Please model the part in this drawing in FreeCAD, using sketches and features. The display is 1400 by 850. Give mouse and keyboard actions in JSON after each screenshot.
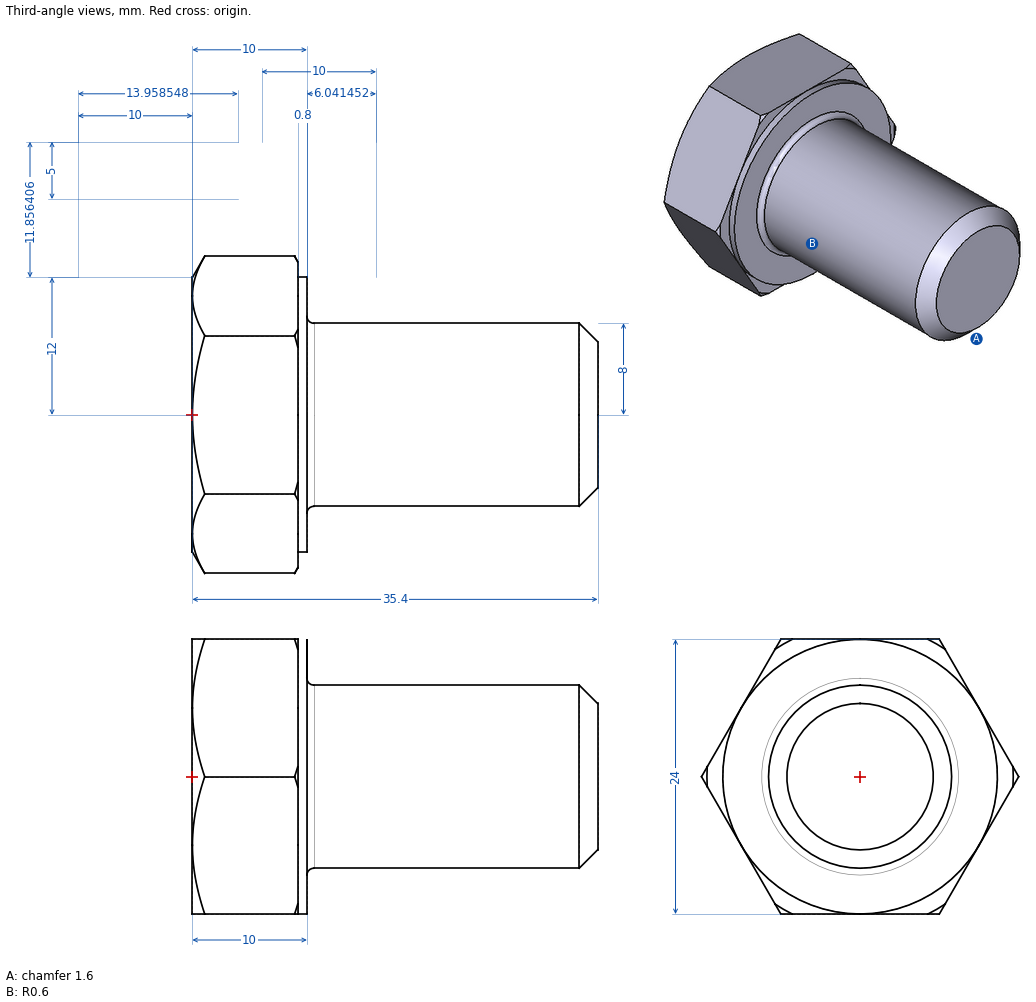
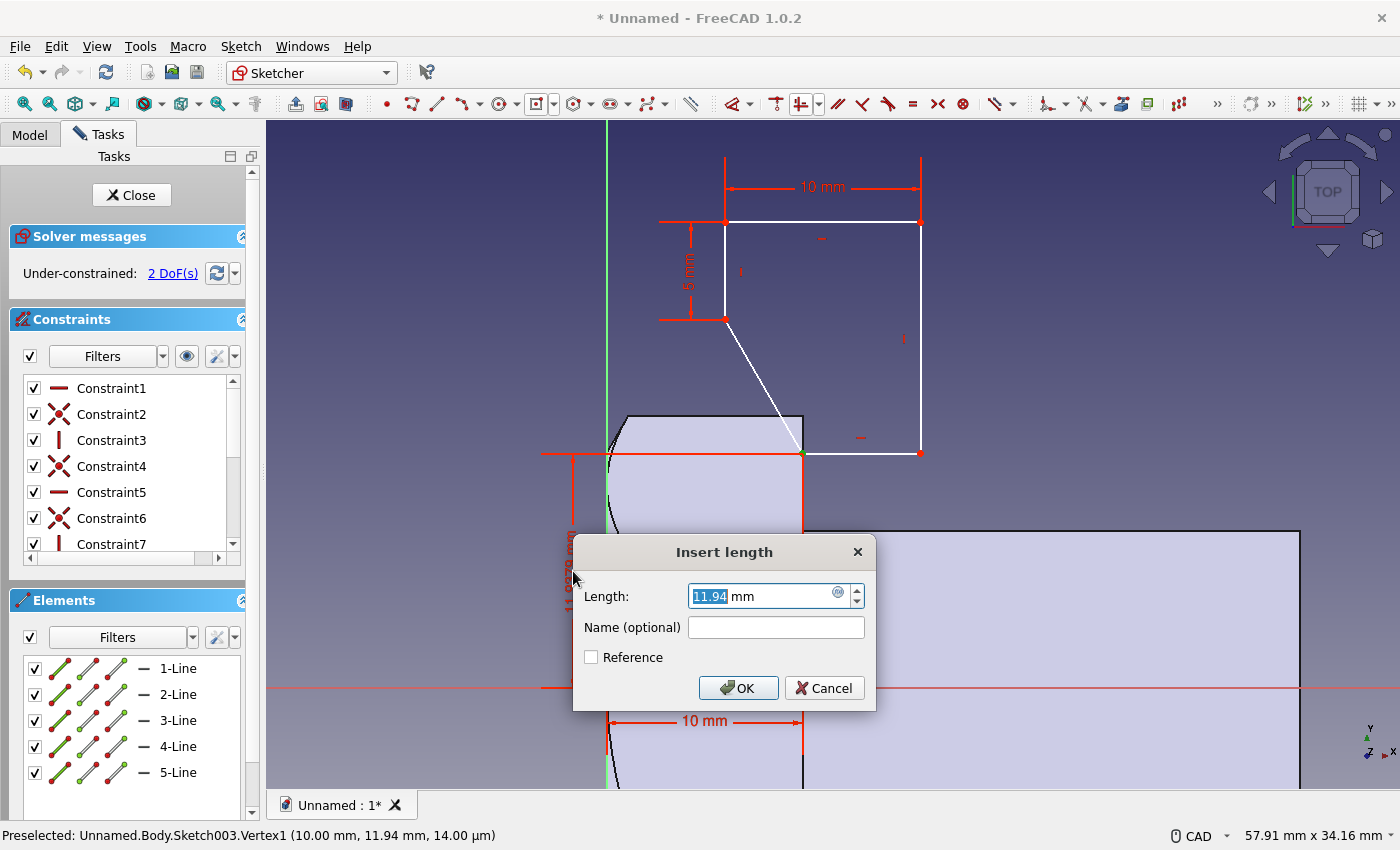
{"action": "type", "text": "12"}
{"action": "key", "text": "Return"}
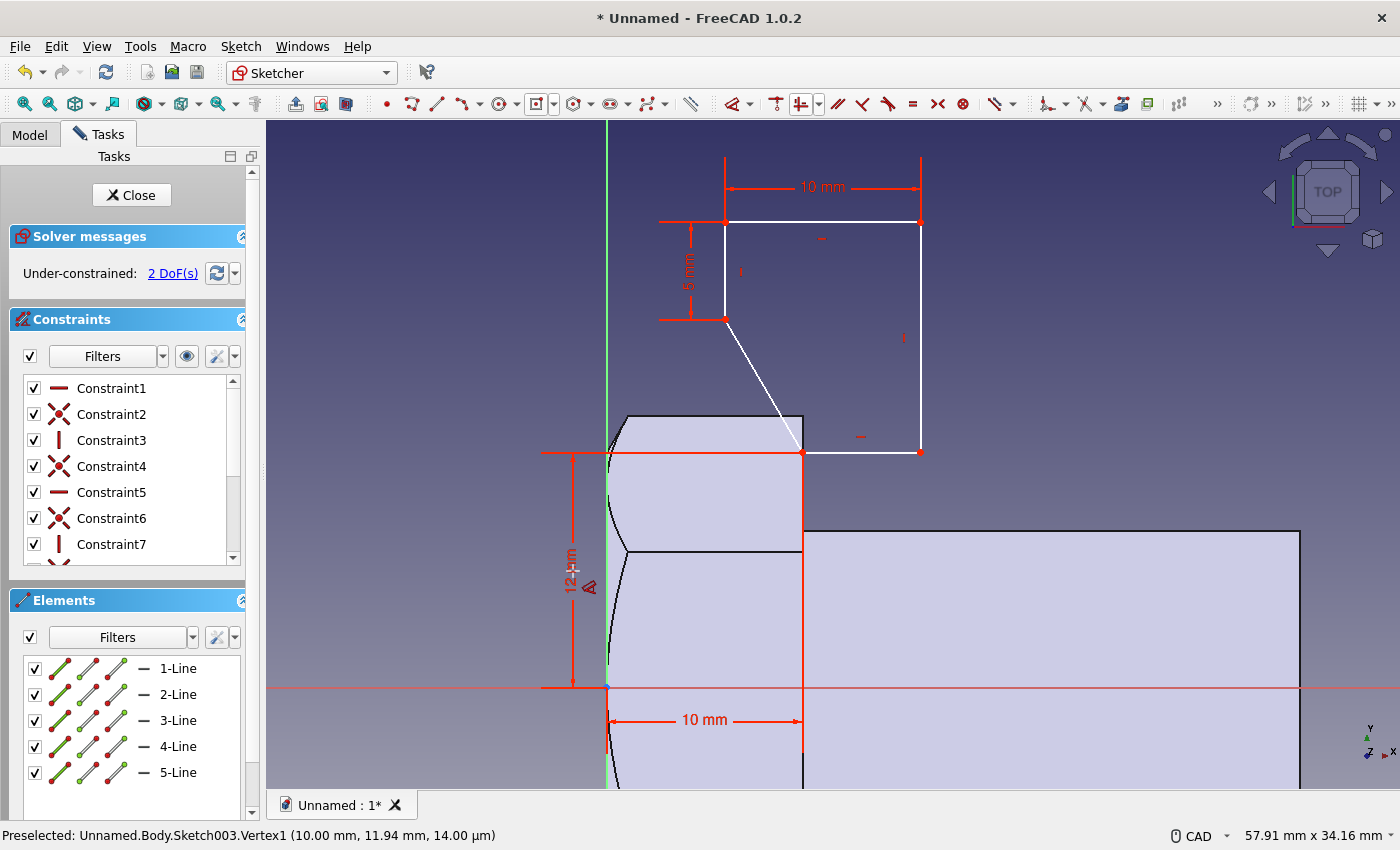
{"action": "left_click", "coordinate": [838, 453]}
{"action": "left_click", "coordinate": [862, 419]}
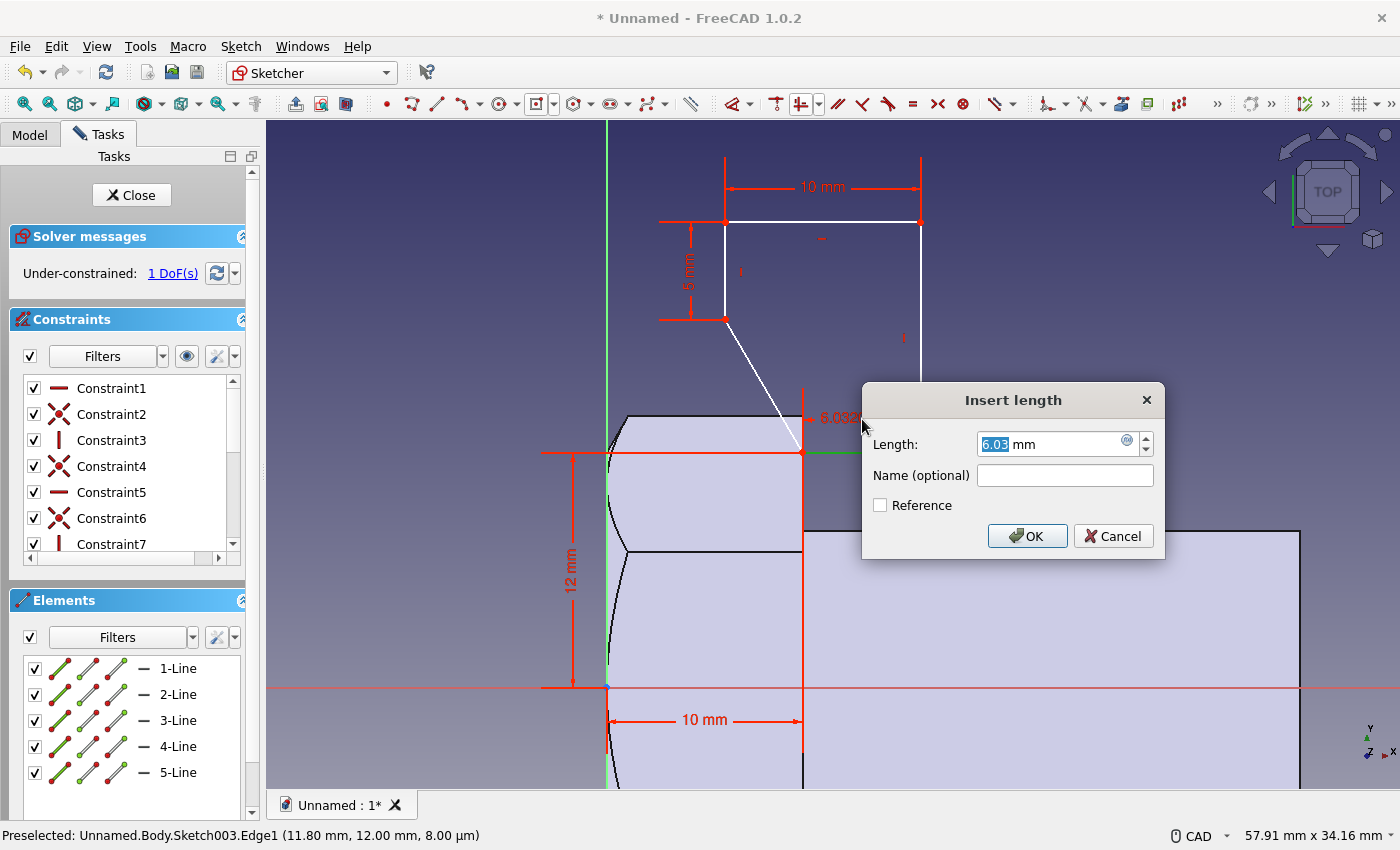
{"action": "type", "text": "6.041452"}
{"action": "key", "text": "Return"}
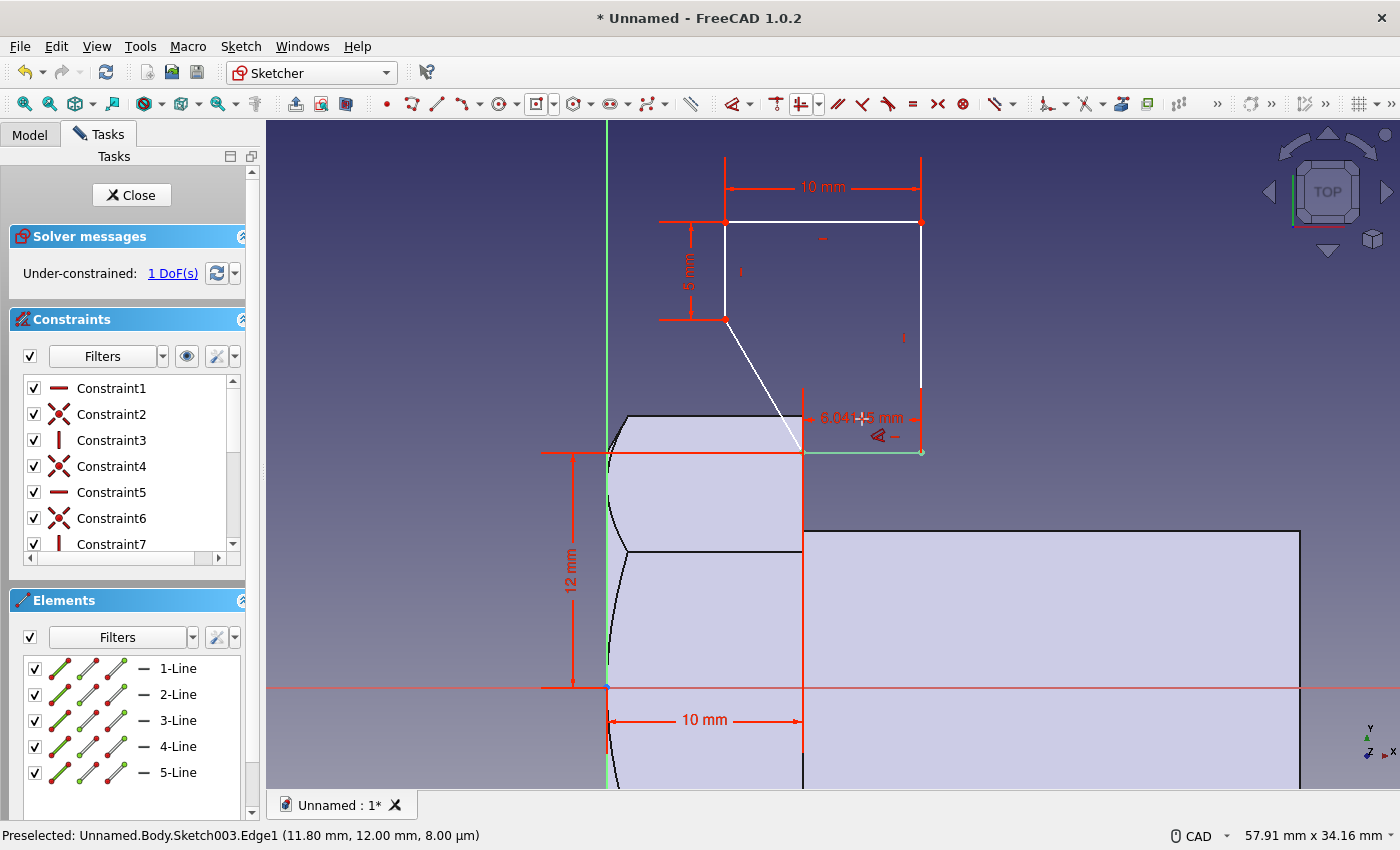
{"action": "left_click", "coordinate": [921, 384]}
{"action": "left_click", "coordinate": [955, 337]}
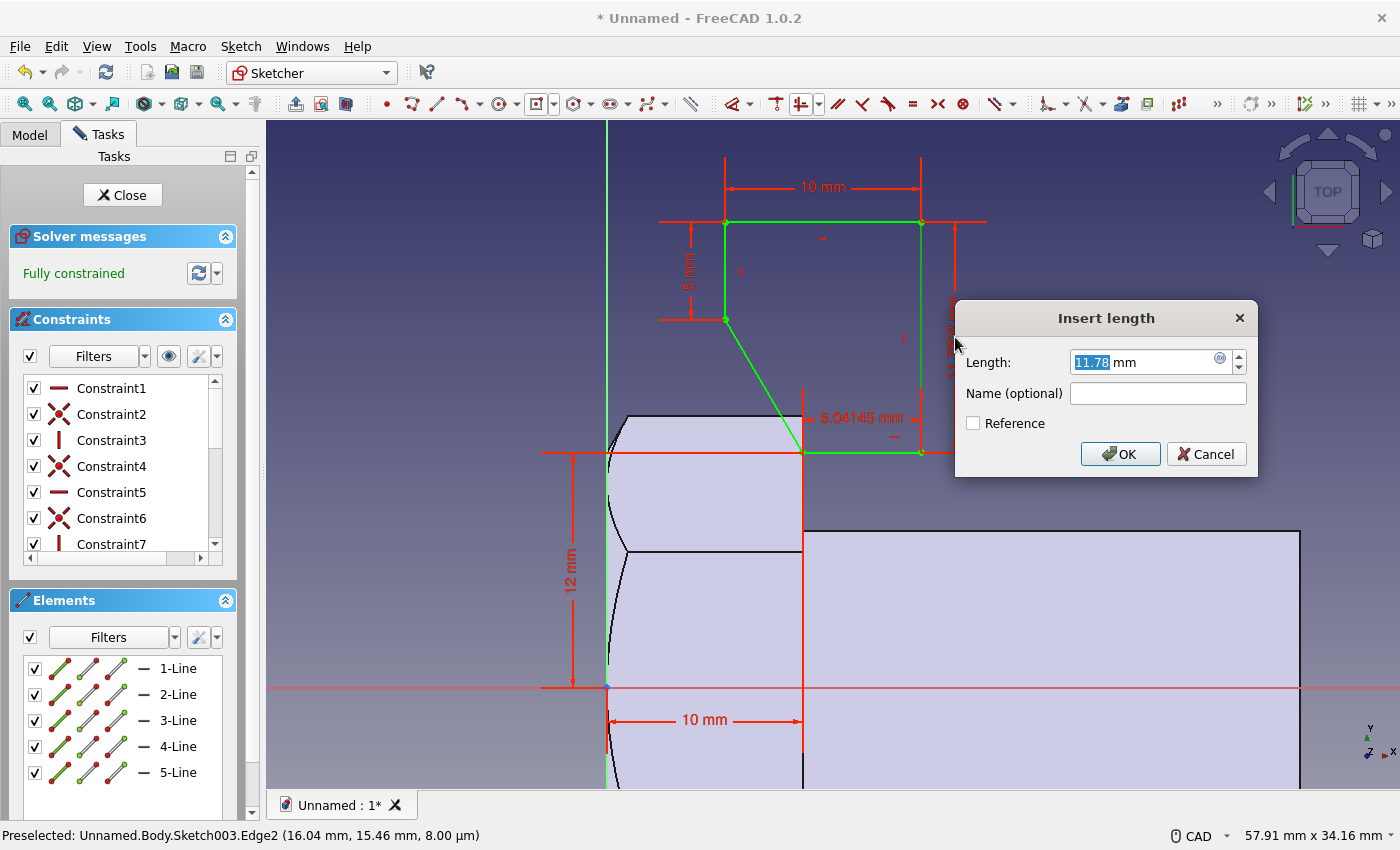
{"action": "type", "text": "11.856406"}
{"action": "key", "text": "Return"}
{"action": "key", "text": "Escape"}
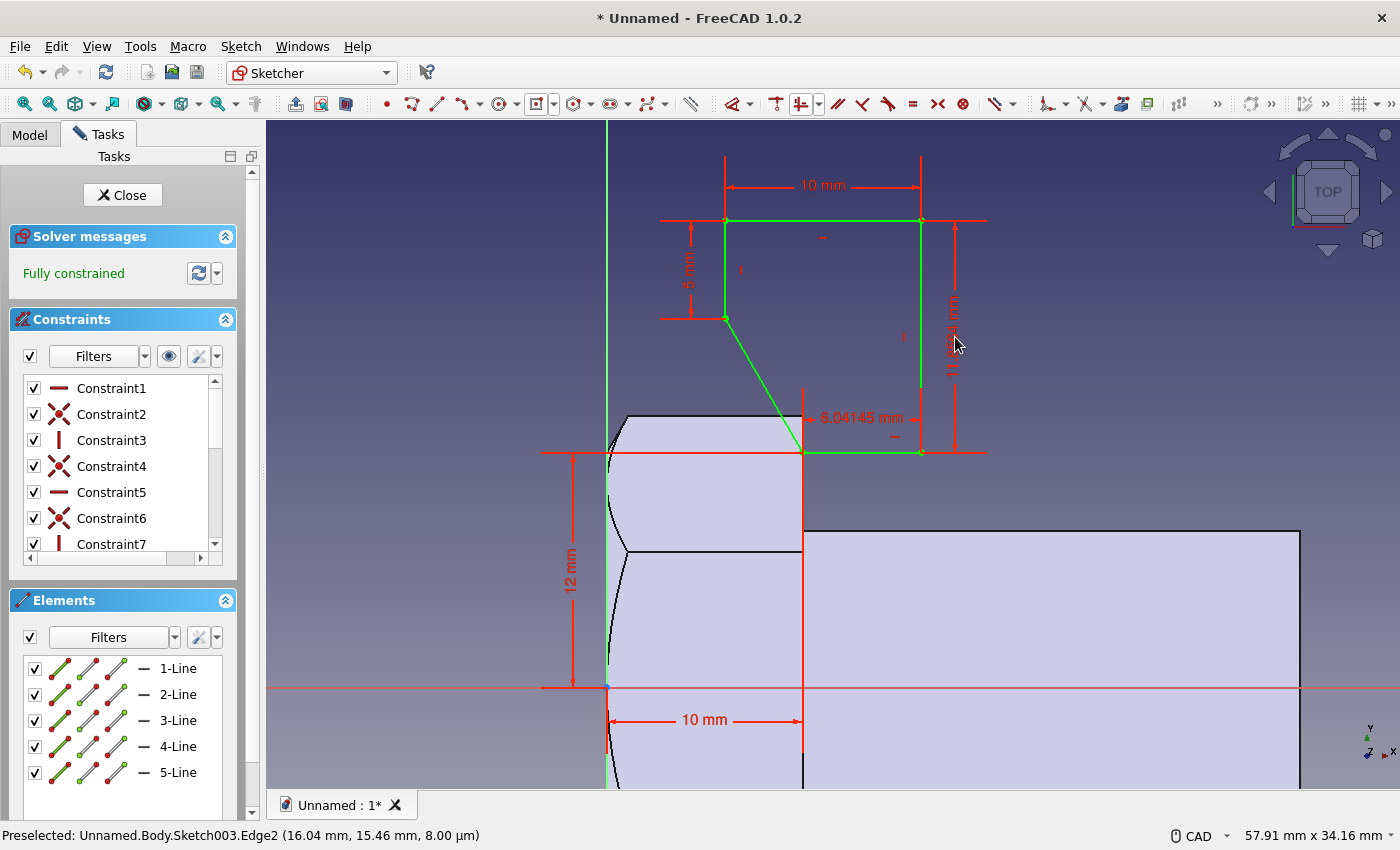
{"action": "left_click", "coordinate": [123, 195]}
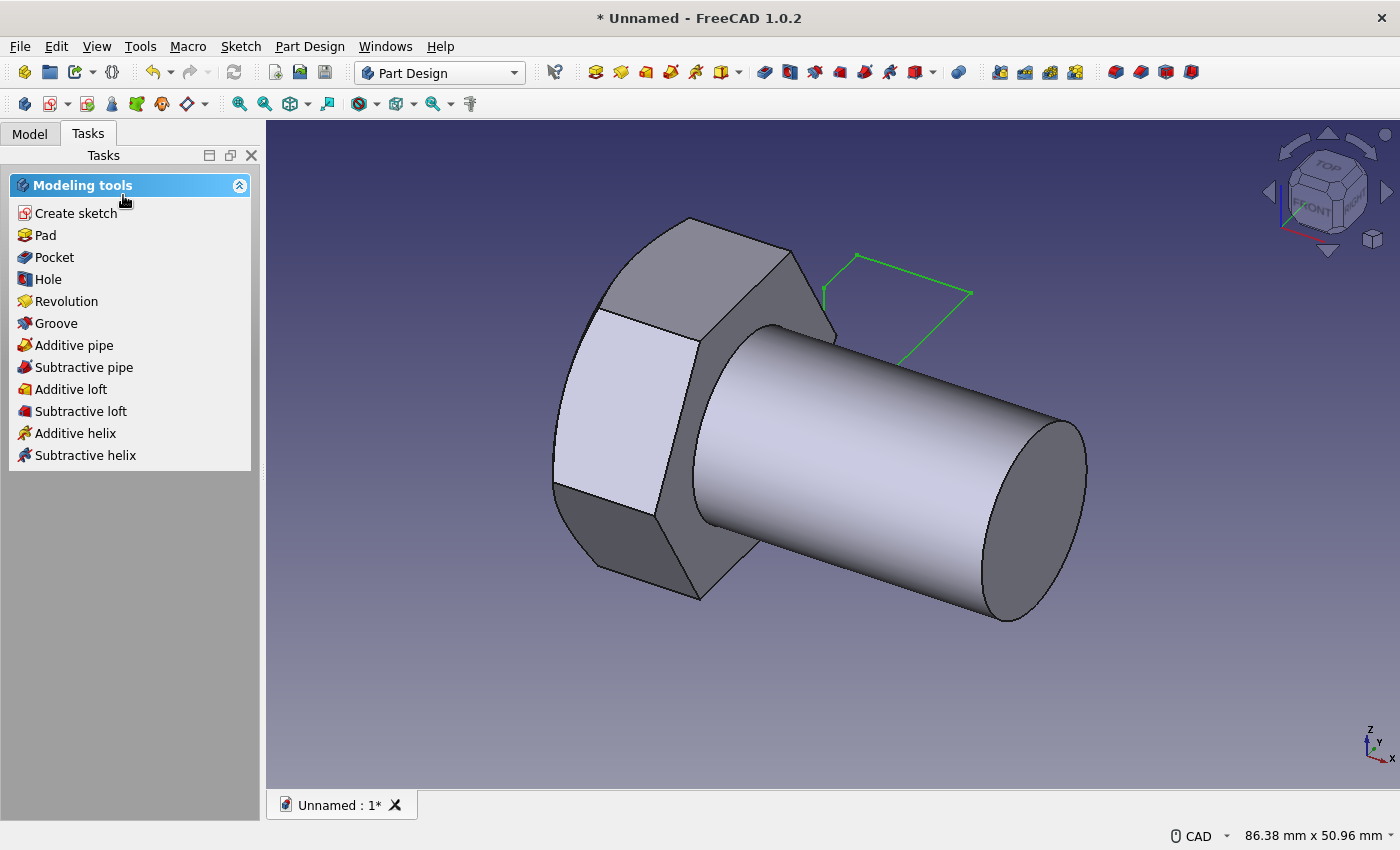
{"action": "left_click", "coordinate": [815, 72]}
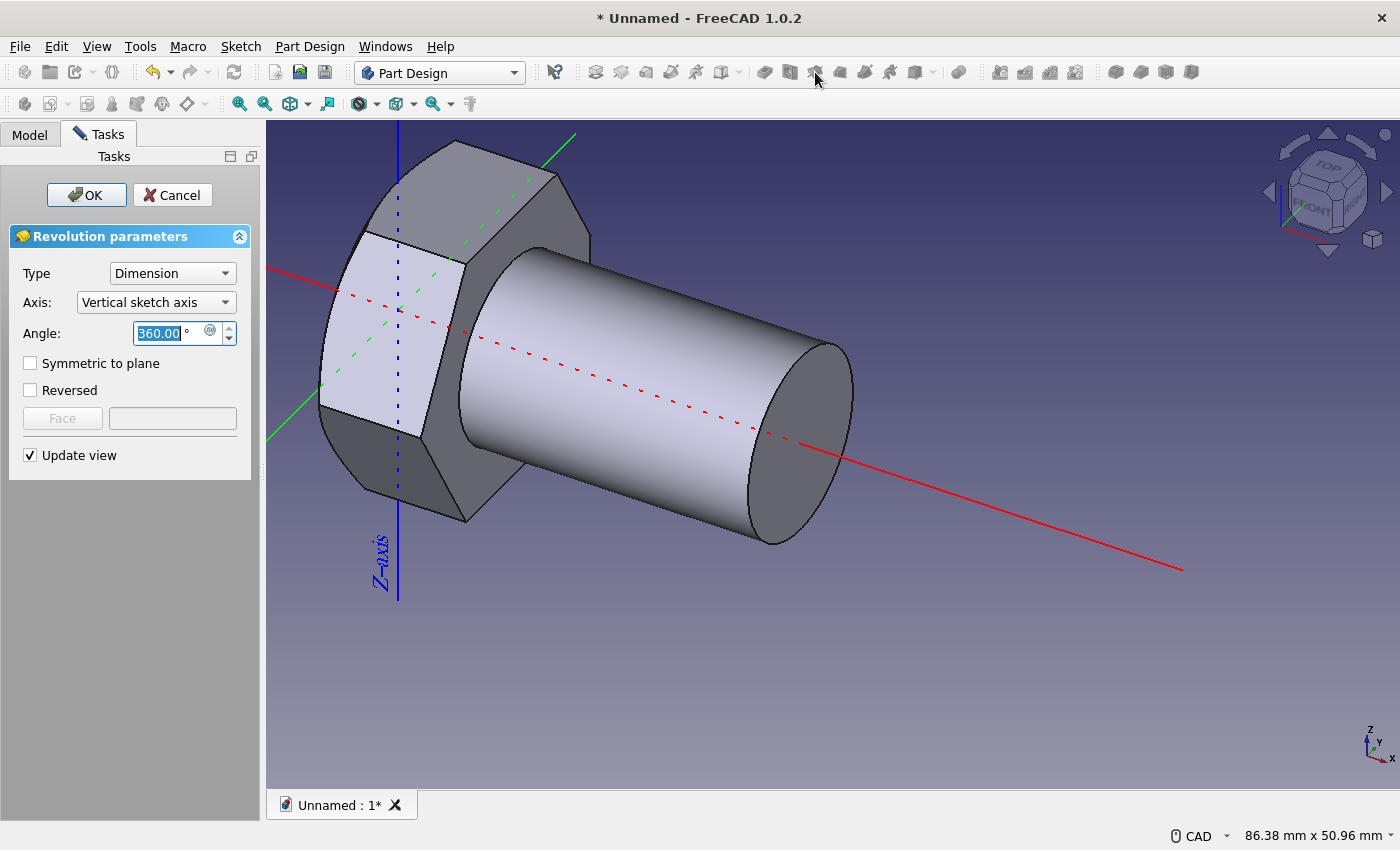
{"action": "left_click", "coordinate": [157, 302]}